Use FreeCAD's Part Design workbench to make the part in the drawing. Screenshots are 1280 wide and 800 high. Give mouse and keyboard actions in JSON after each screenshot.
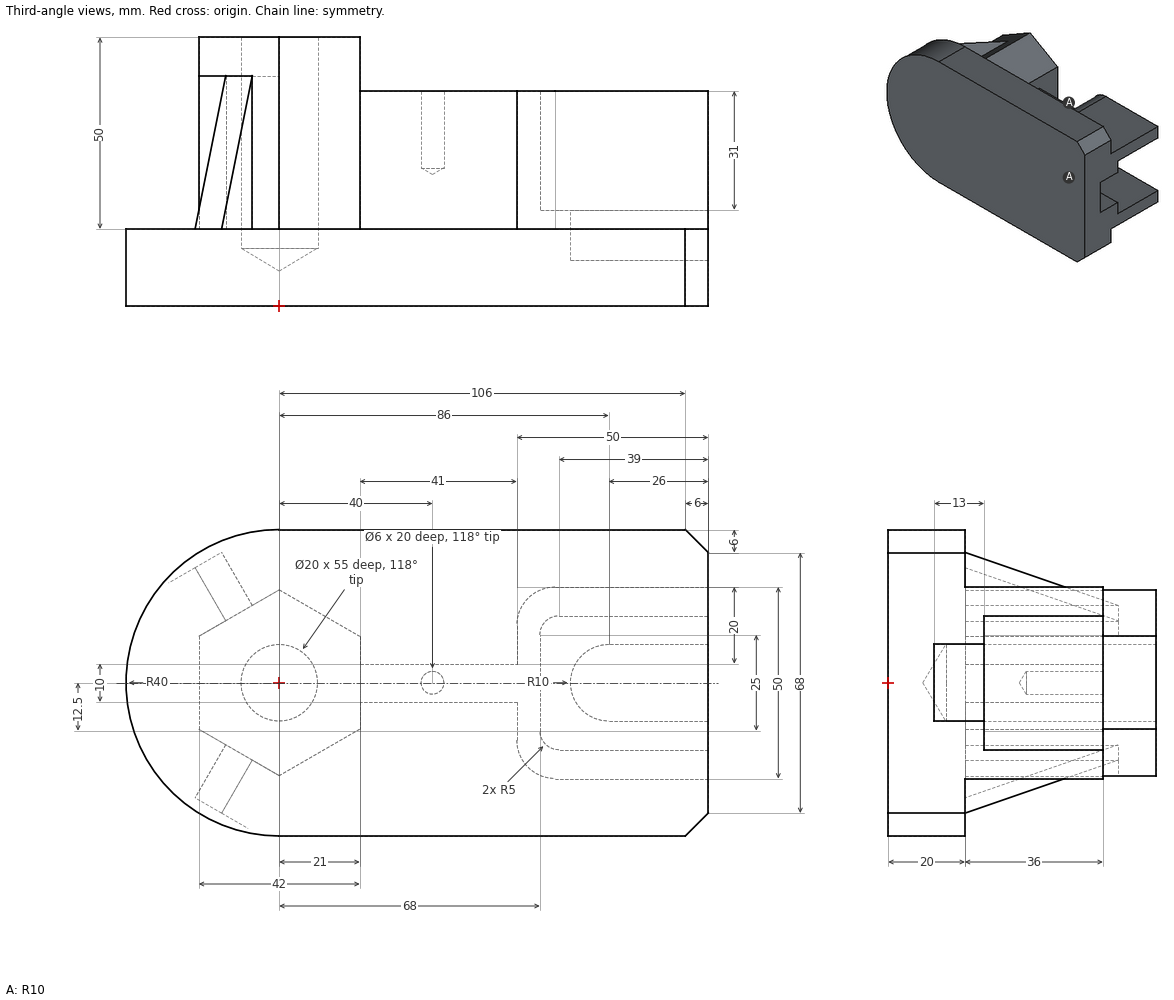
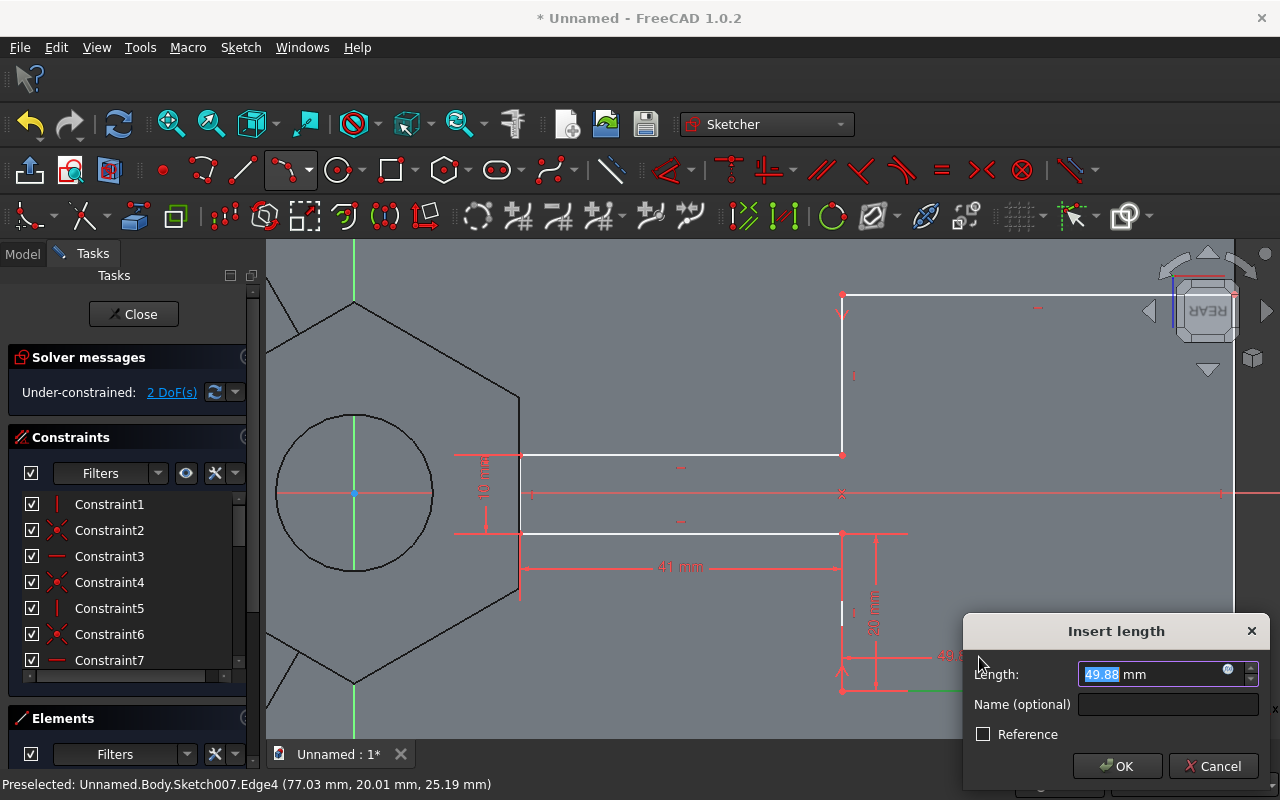
{"action": "type", "text": "50"}
{"action": "key", "text": "Return"}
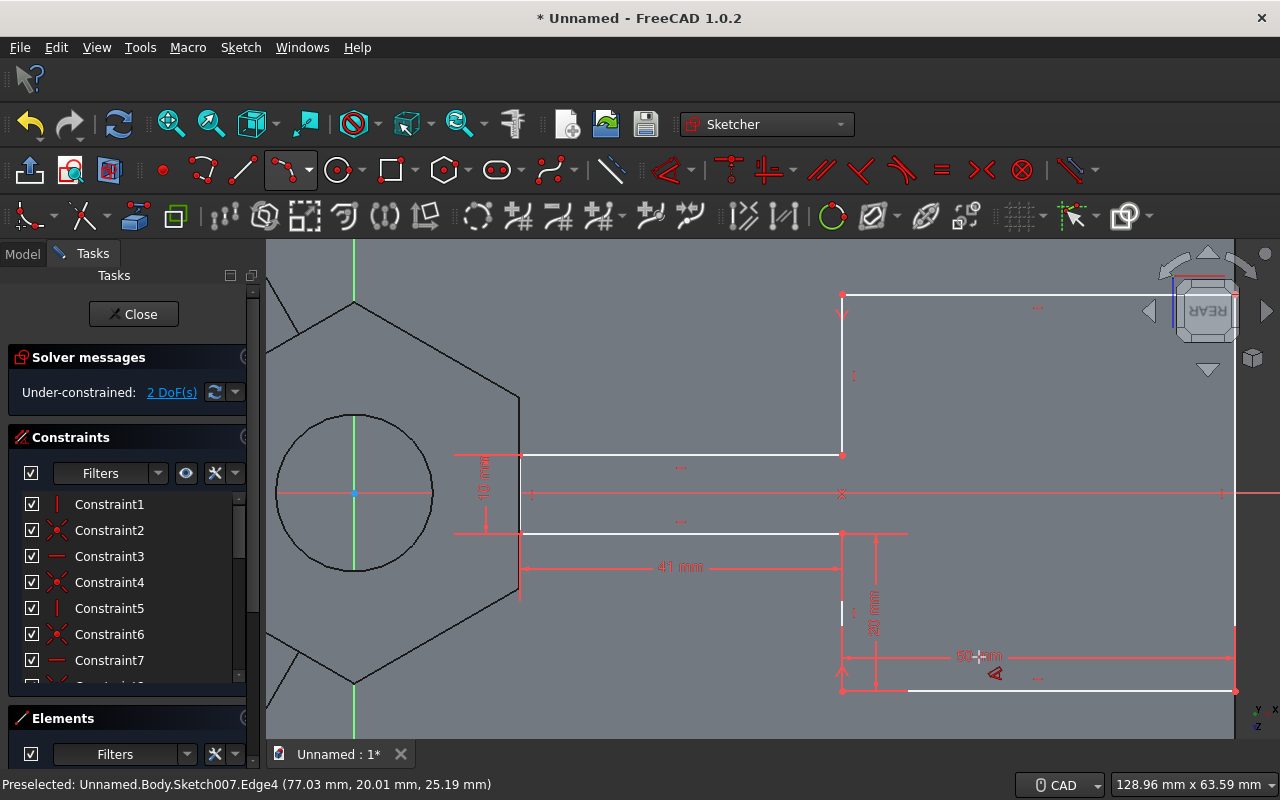
{"action": "scroll", "coordinate": [521, 481], "scroll_direction": "down", "scroll_amount": 2}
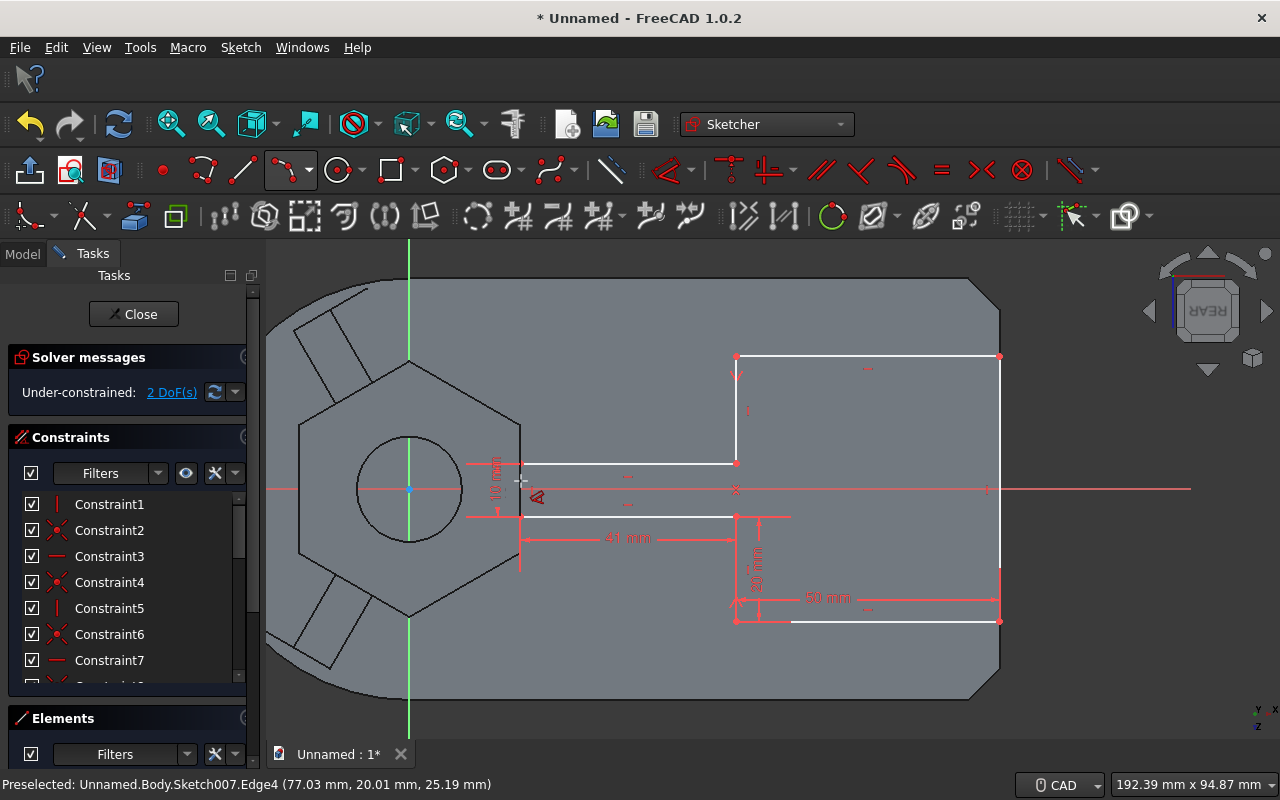
{"action": "left_click", "coordinate": [1000, 542]}
{"action": "left_click", "coordinate": [1034, 428]}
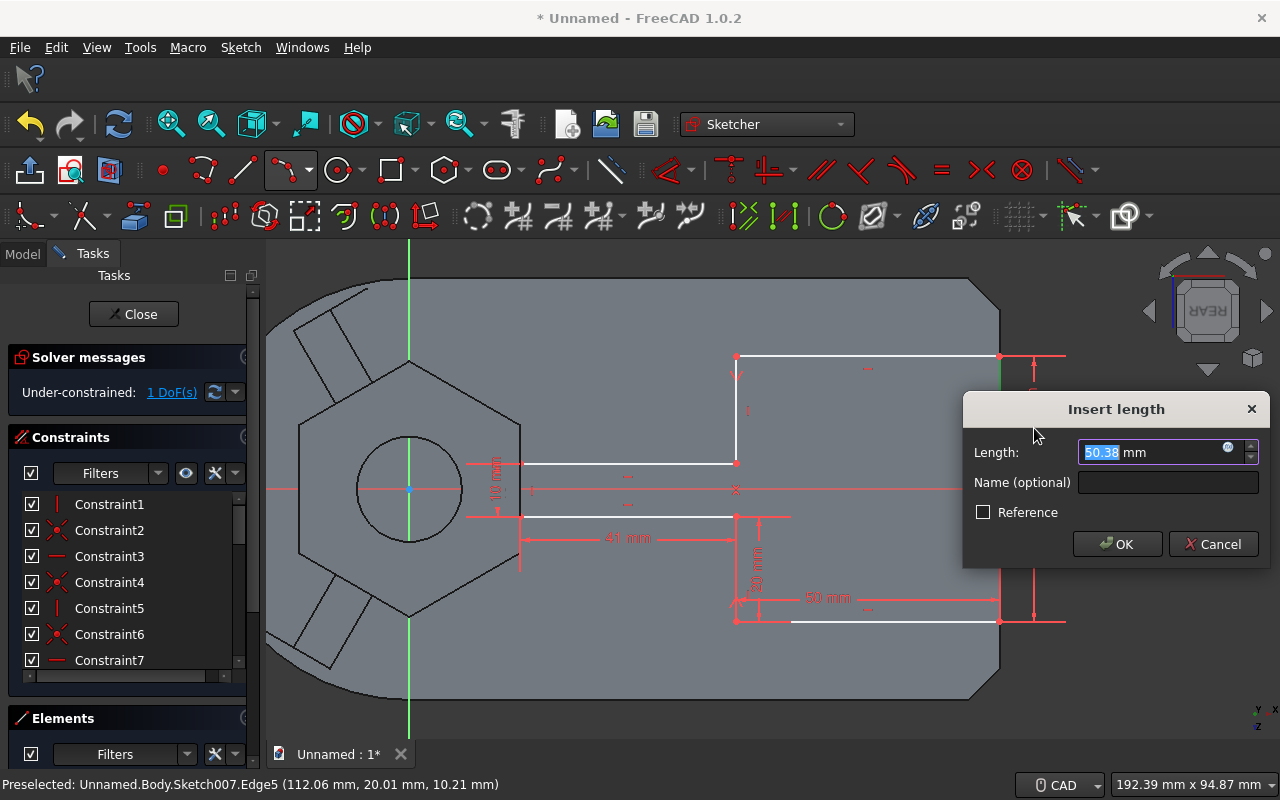
{"action": "type", "text": "50"}
{"action": "key", "text": "Return"}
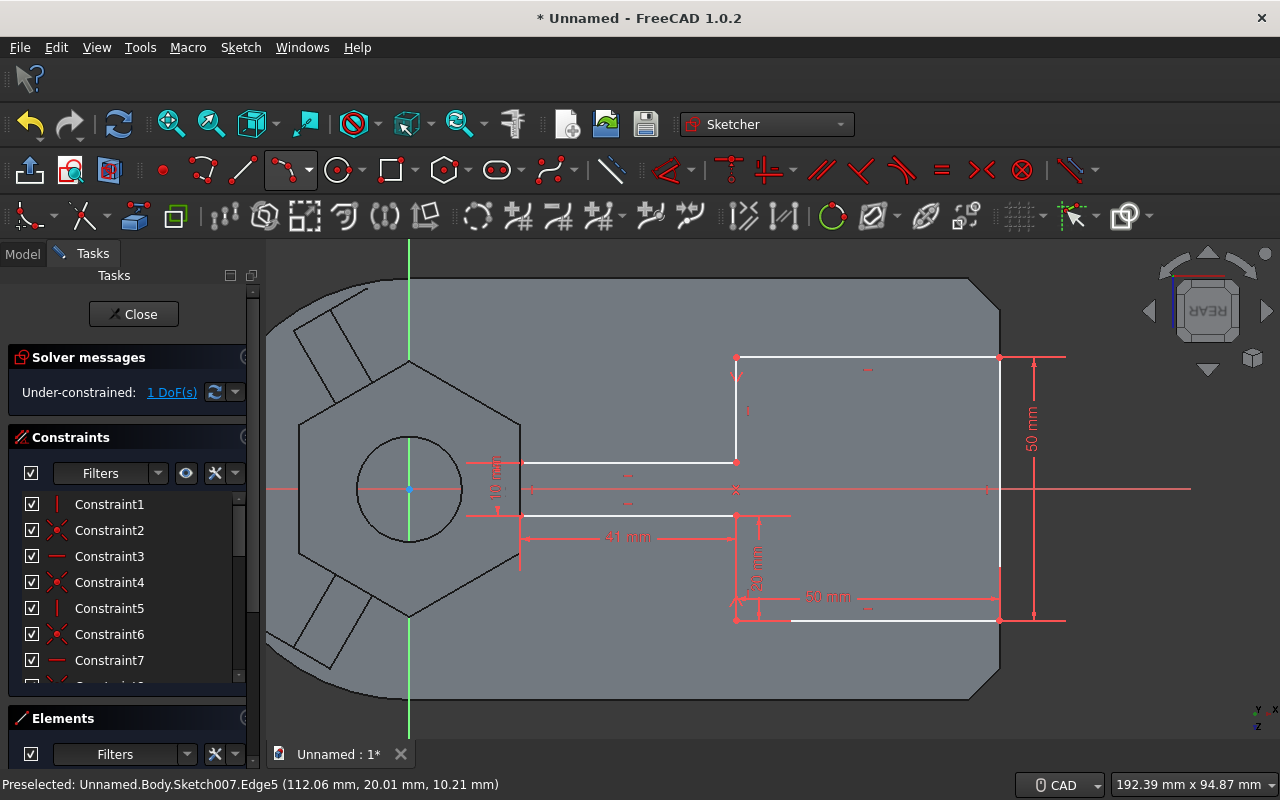
{"action": "left_click", "coordinate": [520, 463]}
{"action": "left_click", "coordinate": [465, 429]}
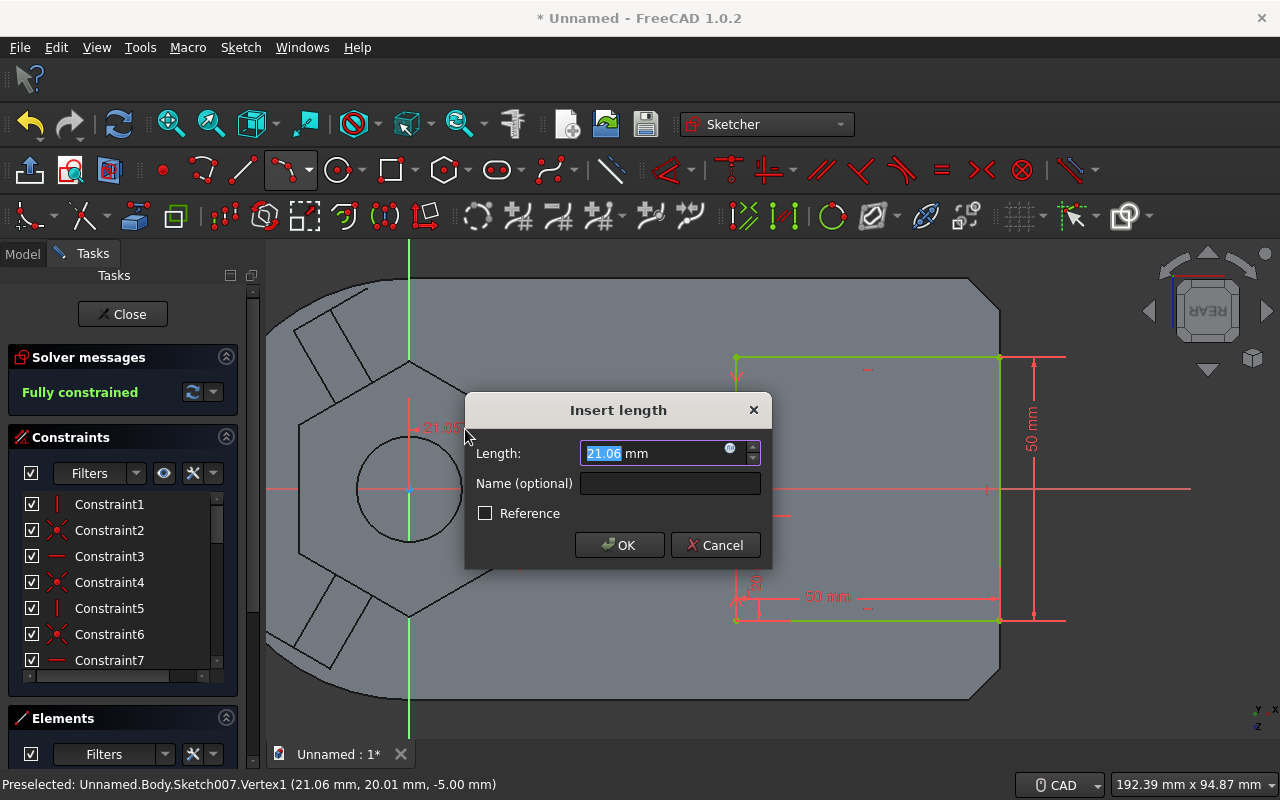
{"action": "type", "text": "21"}
{"action": "key", "text": "Return"}
{"action": "key", "text": "Escape"}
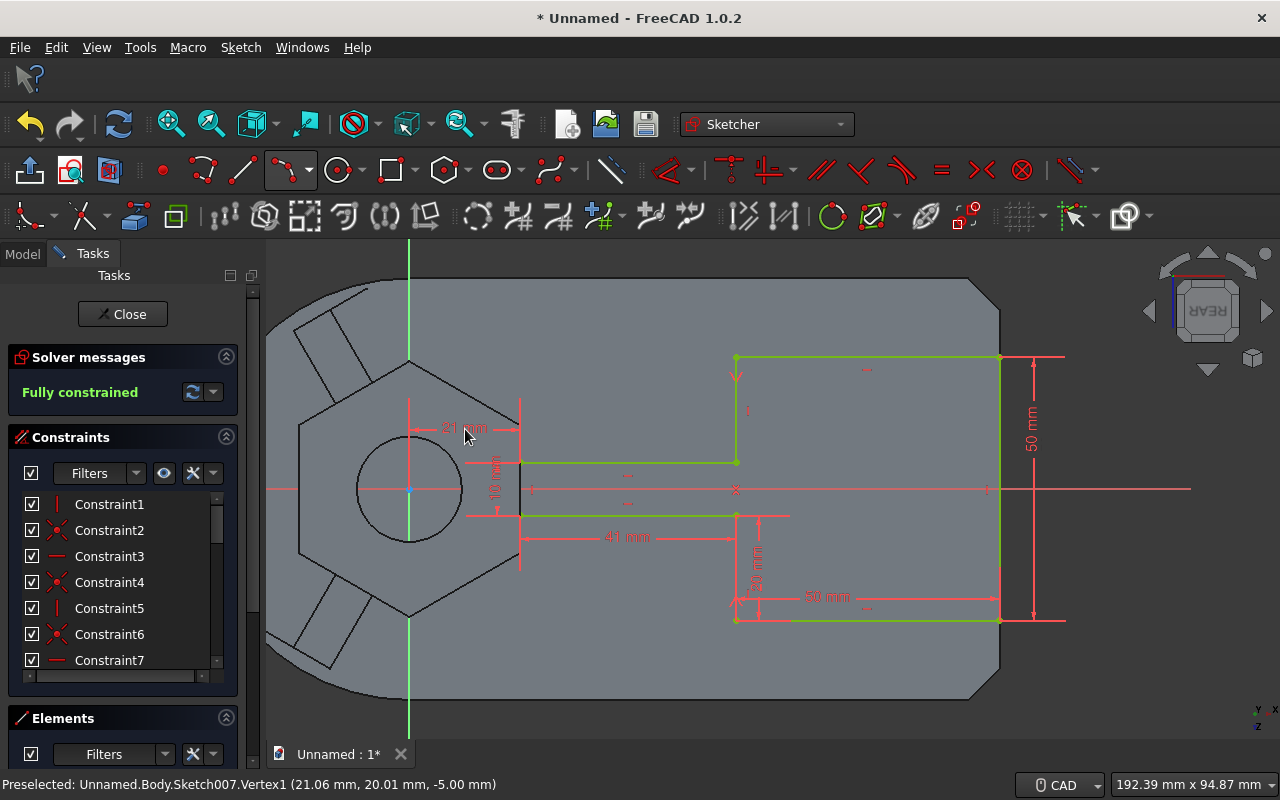
{"action": "left_click", "coordinate": [123, 314]}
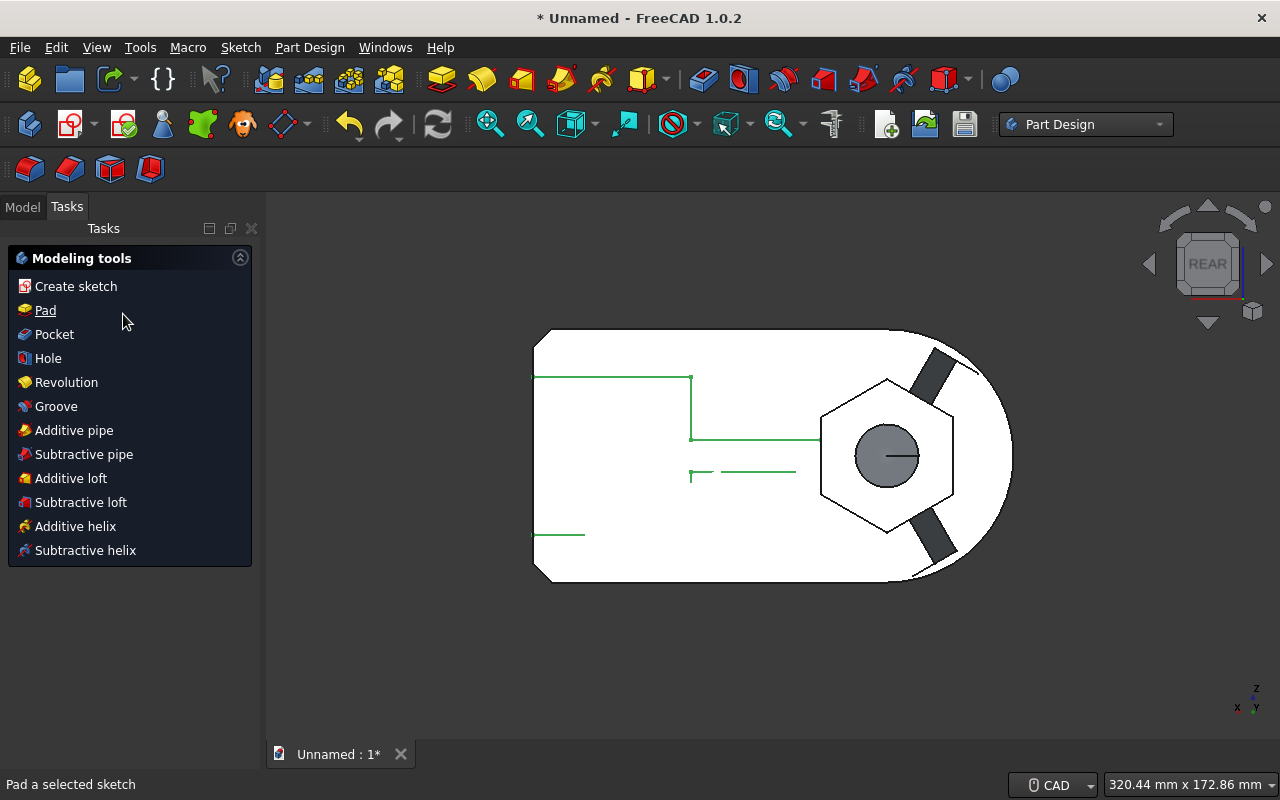
{"action": "left_click", "coordinate": [442, 80]}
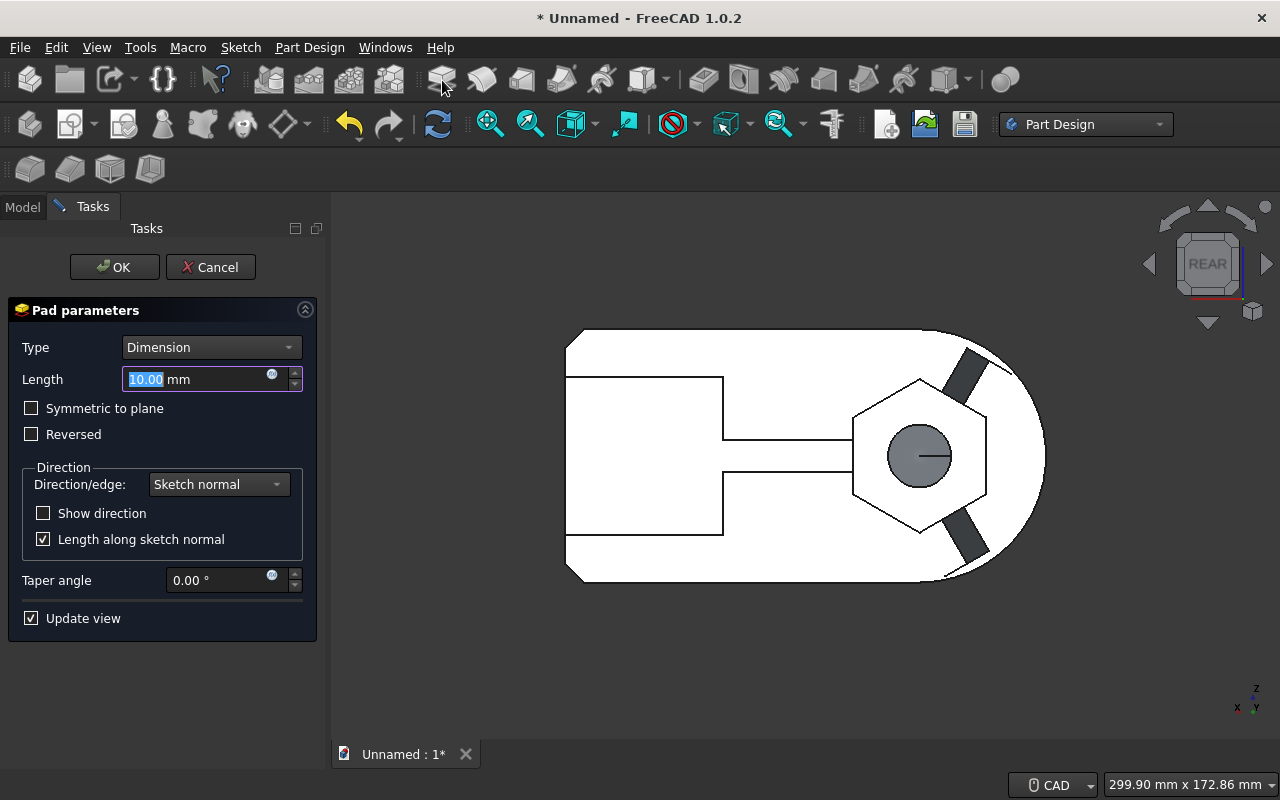
{"action": "type", "text": "36"}
{"action": "key", "text": "Tab"}